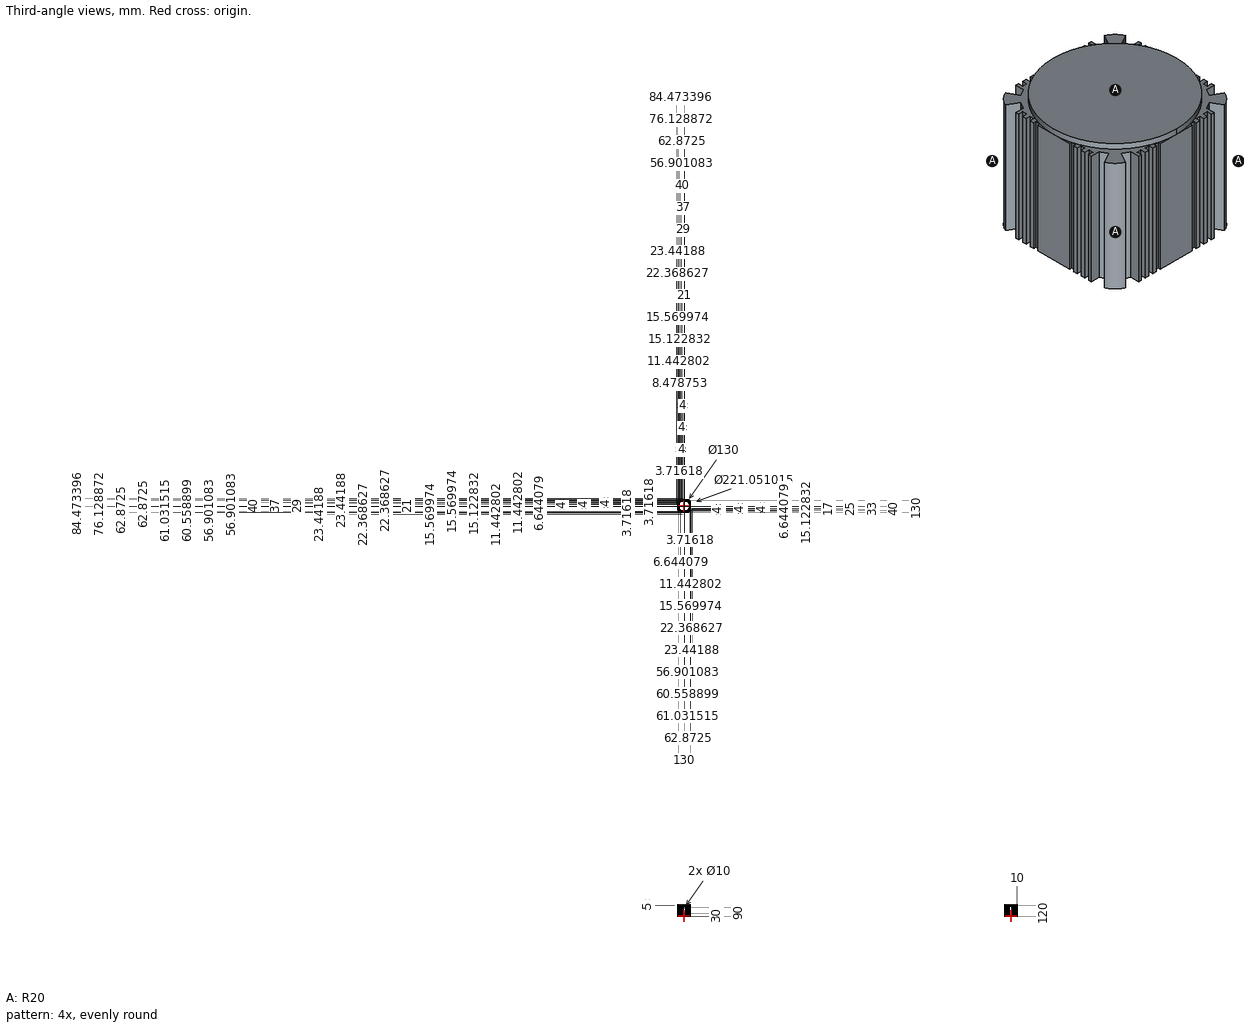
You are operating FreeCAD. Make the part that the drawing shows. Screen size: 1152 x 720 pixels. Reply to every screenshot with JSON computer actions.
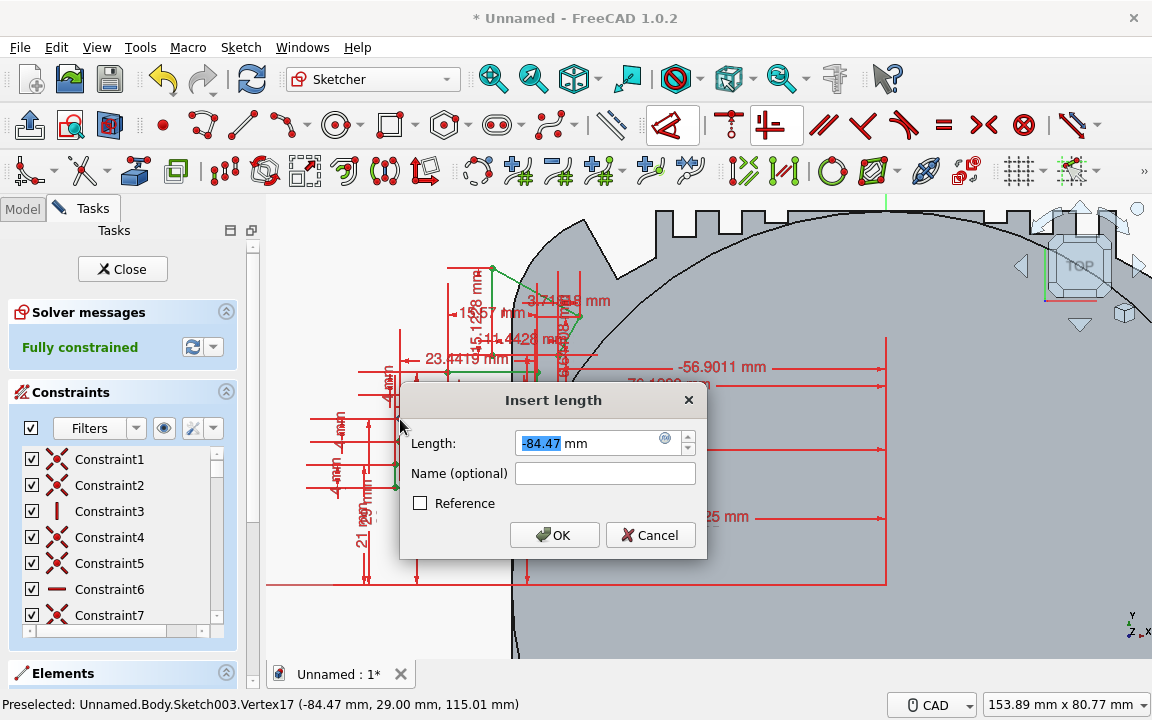
{"action": "type", "text": "-84.473396"}
{"action": "key", "text": "Return"}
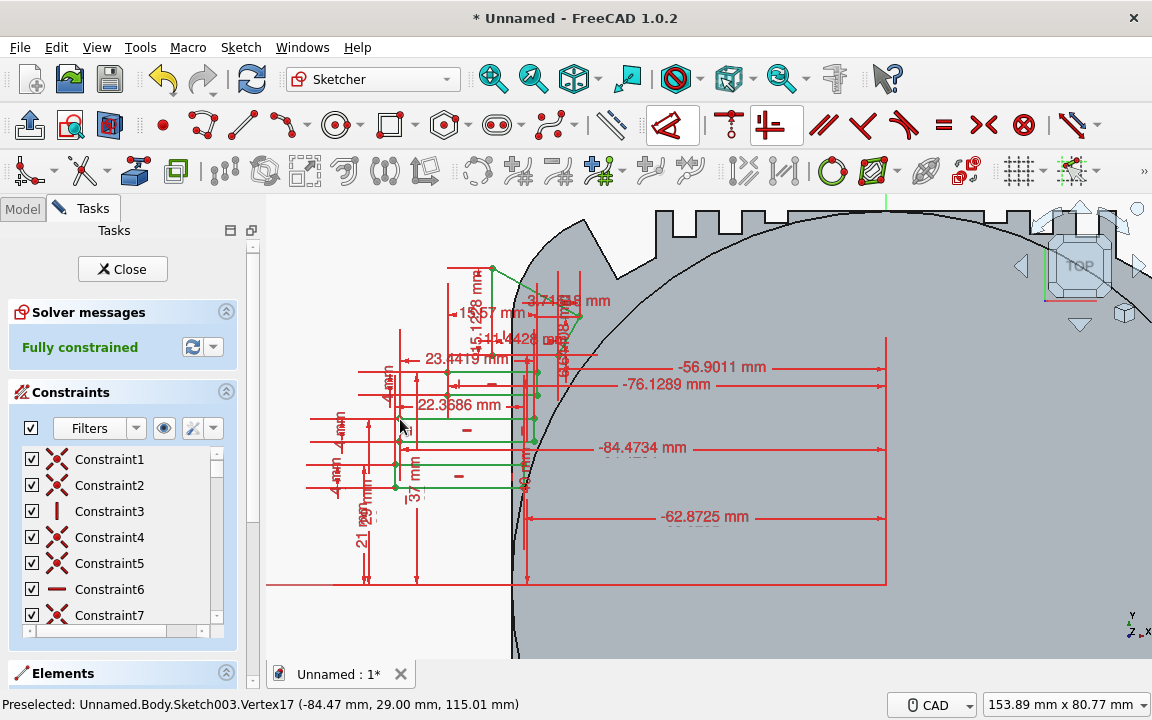
{"action": "left_click", "coordinate": [123, 269]}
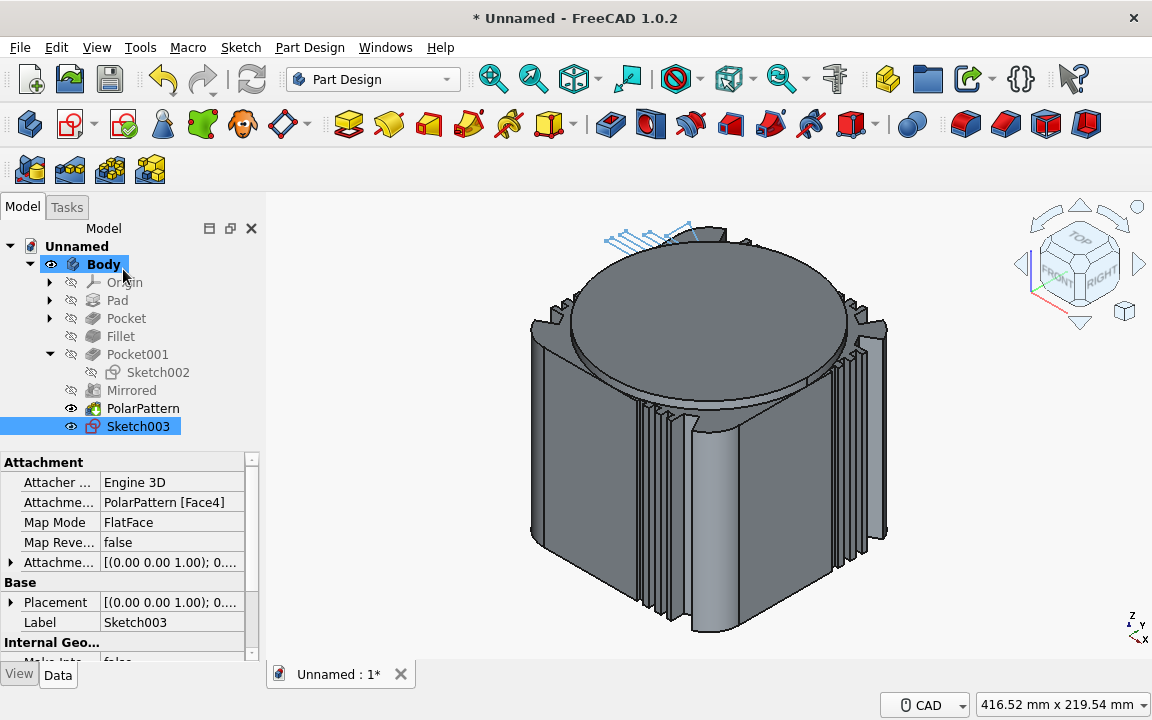
{"action": "left_click", "coordinate": [612, 124]}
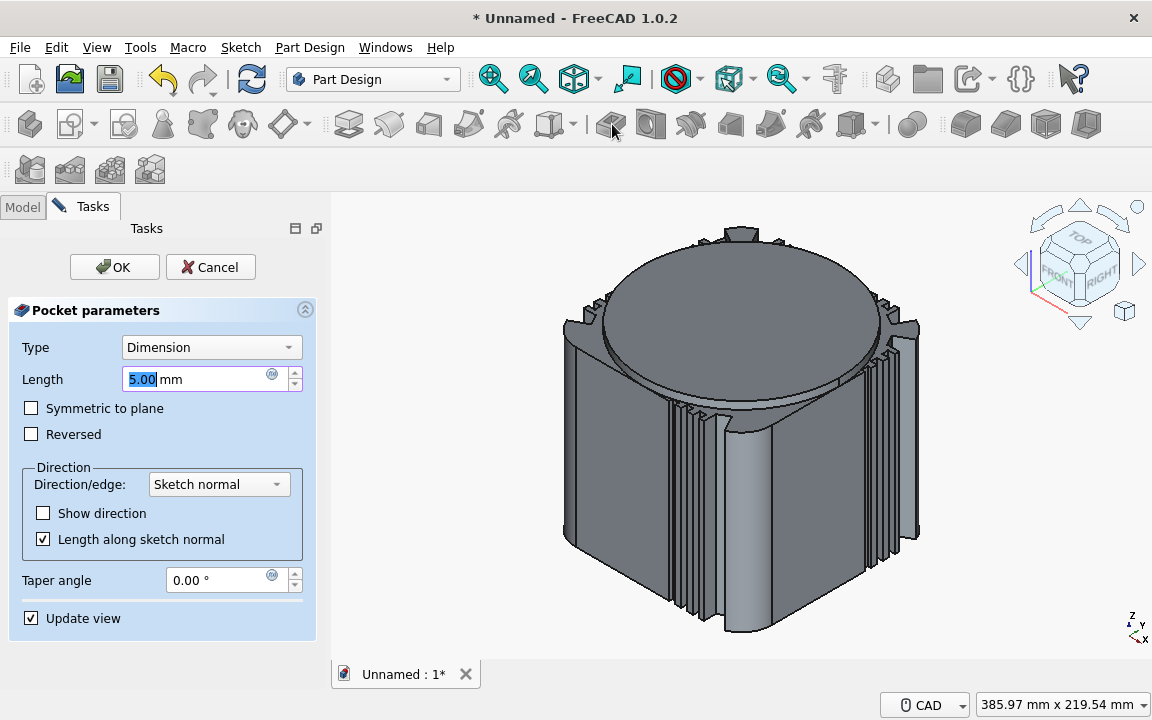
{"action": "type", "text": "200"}
{"action": "key", "text": "Tab"}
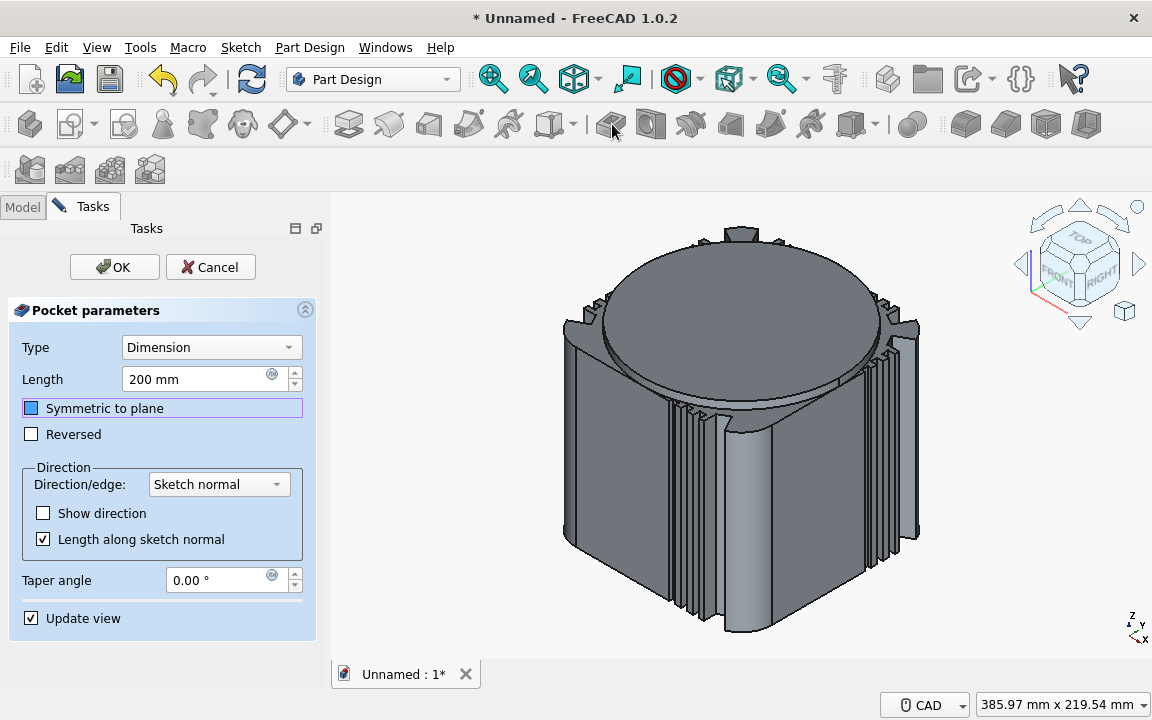
{"action": "left_click", "coordinate": [115, 267]}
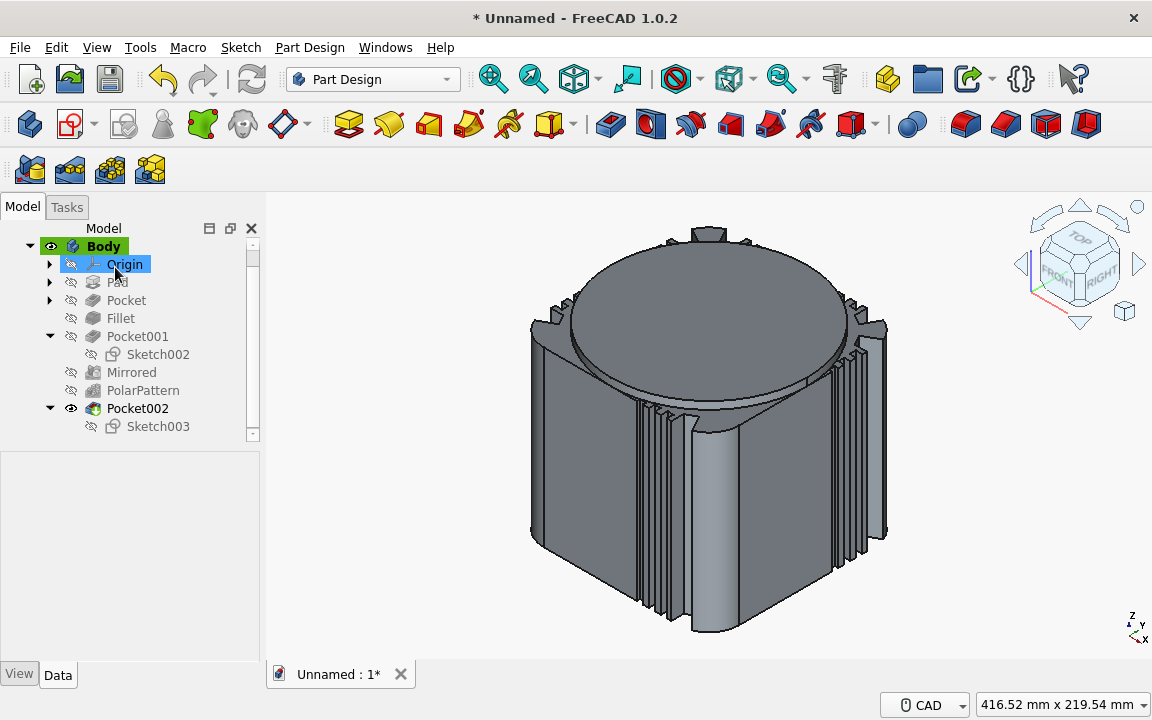
{"action": "left_click", "coordinate": [709, 418]}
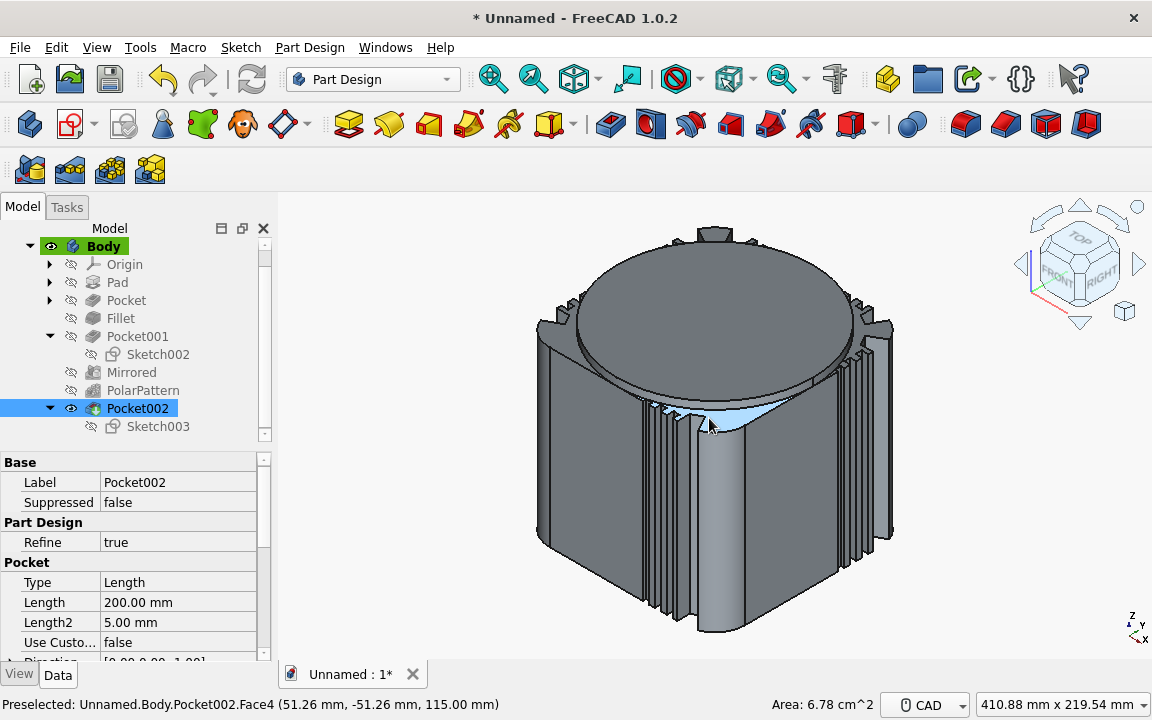
{"action": "left_click", "coordinate": [70, 124]}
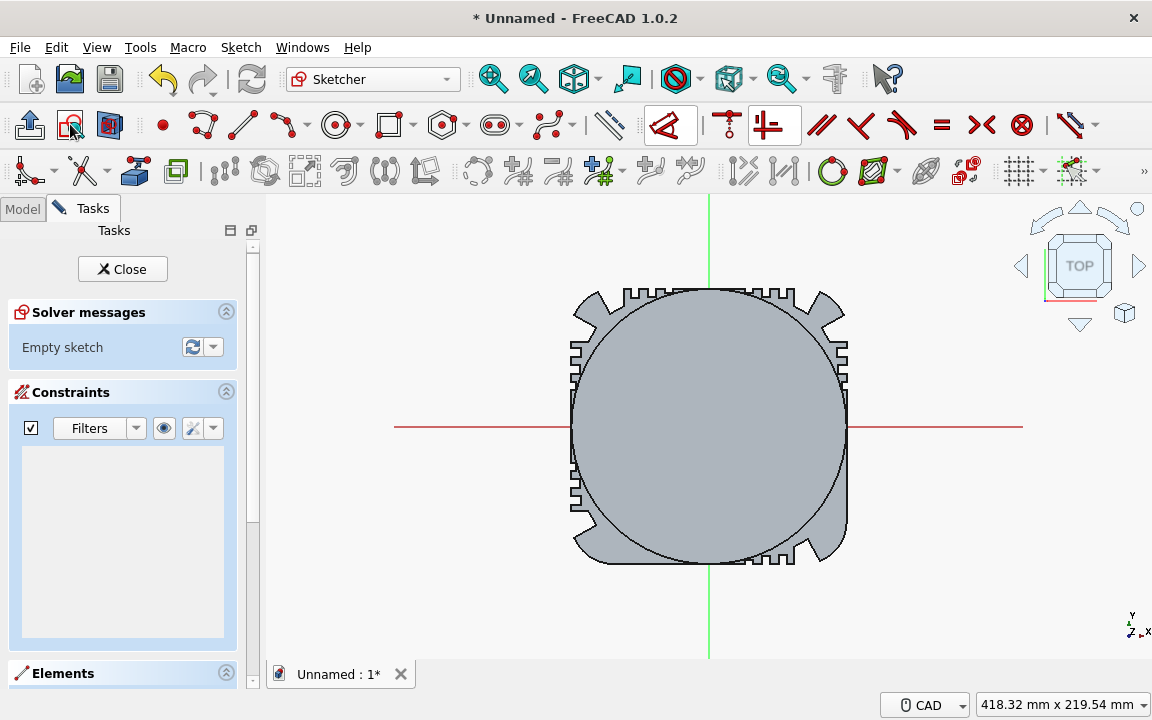
{"action": "scroll", "coordinate": [671, 631], "scroll_direction": "up", "scroll_amount": 2}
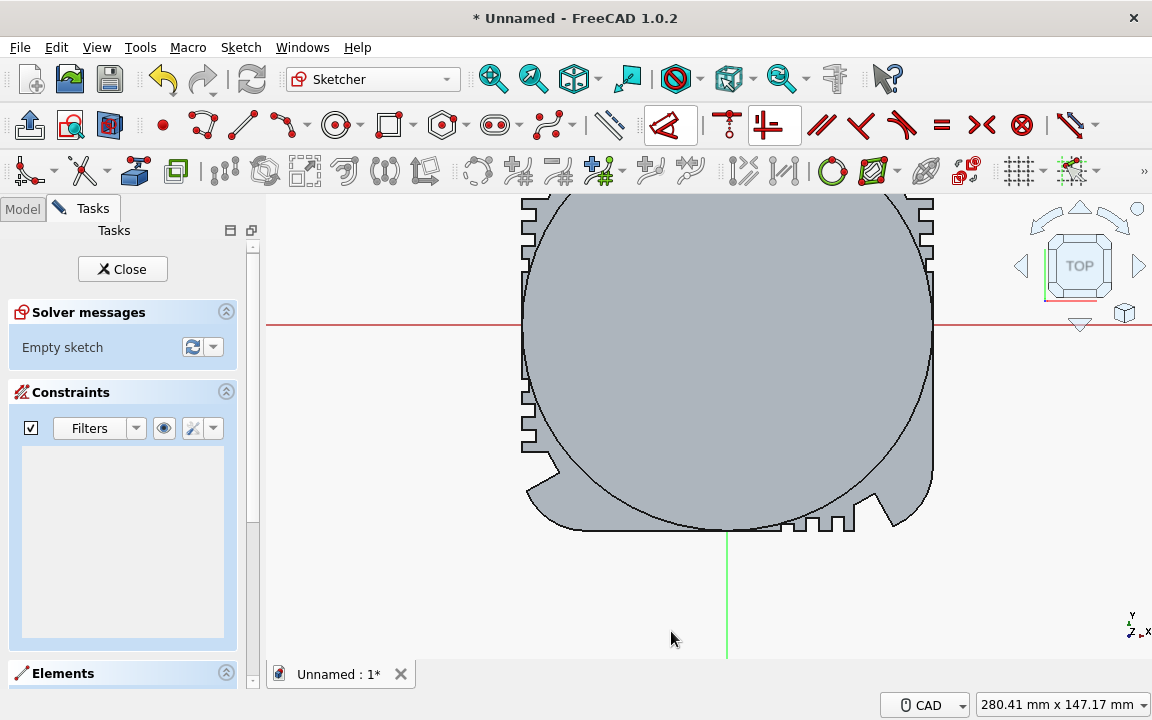
{"action": "left_click", "coordinate": [204, 126]}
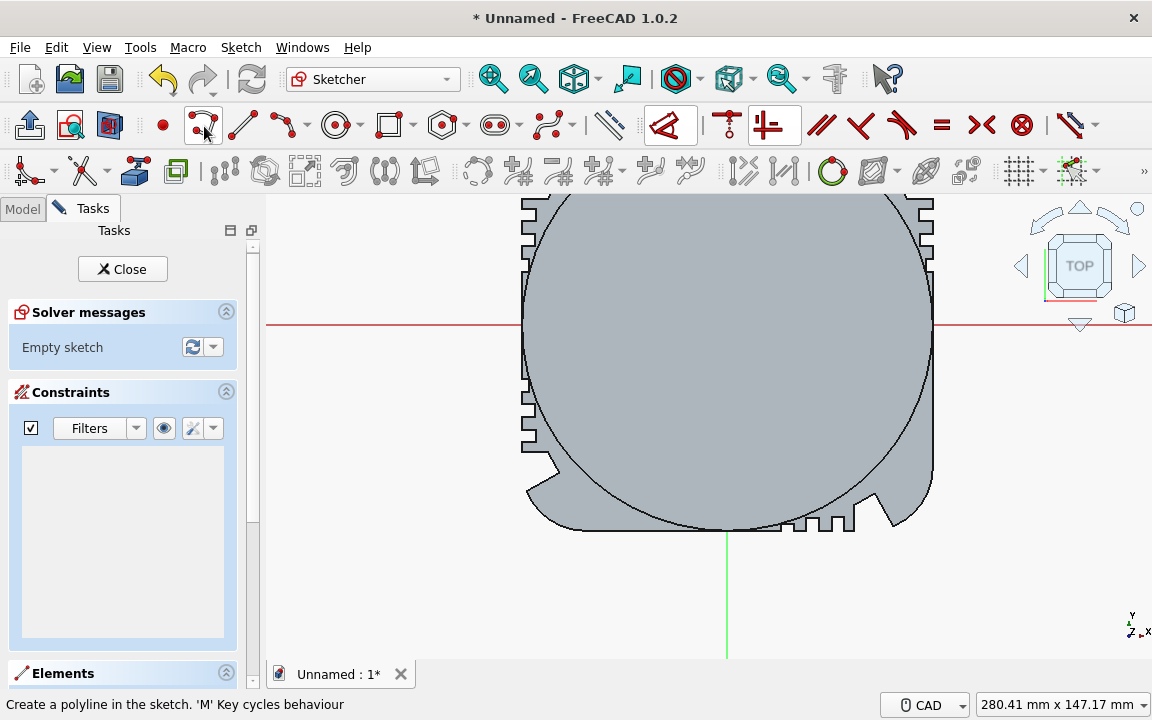
{"action": "left_click", "coordinate": [601, 505]}
{"action": "left_click", "coordinate": [580, 494]}
{"action": "left_click", "coordinate": [553, 541]}
{"action": "left_click", "coordinate": [601, 541]}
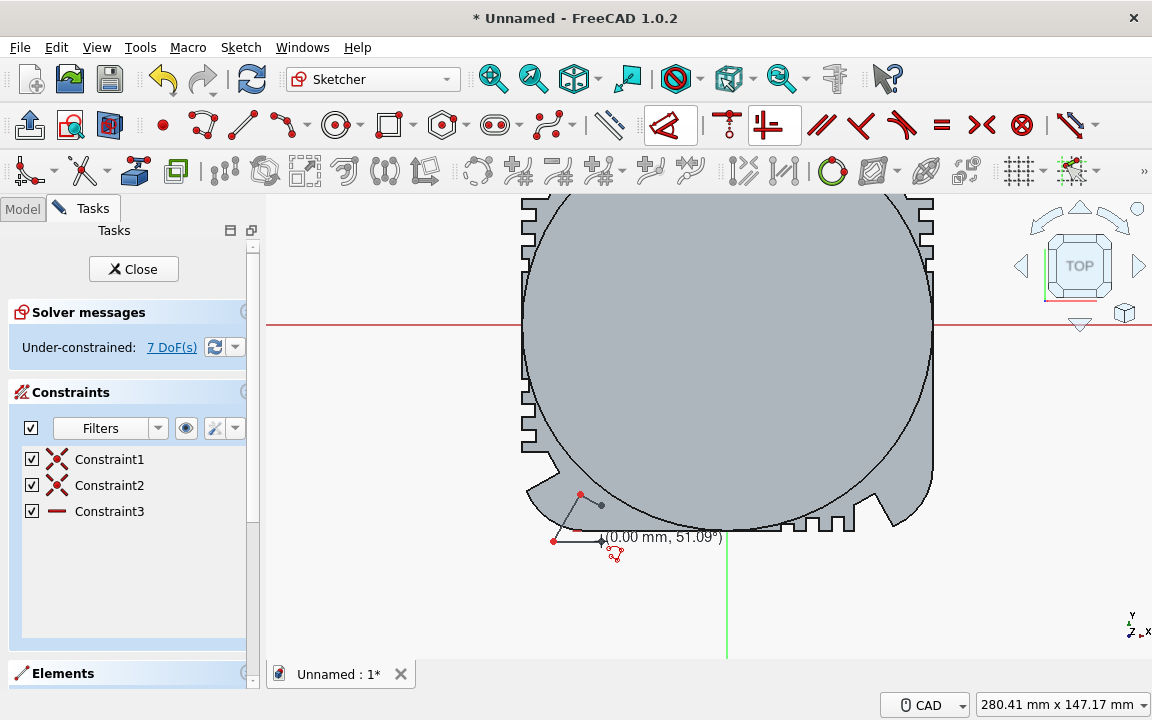
{"action": "scroll", "coordinate": [601, 505], "scroll_direction": "up", "scroll_amount": 2}